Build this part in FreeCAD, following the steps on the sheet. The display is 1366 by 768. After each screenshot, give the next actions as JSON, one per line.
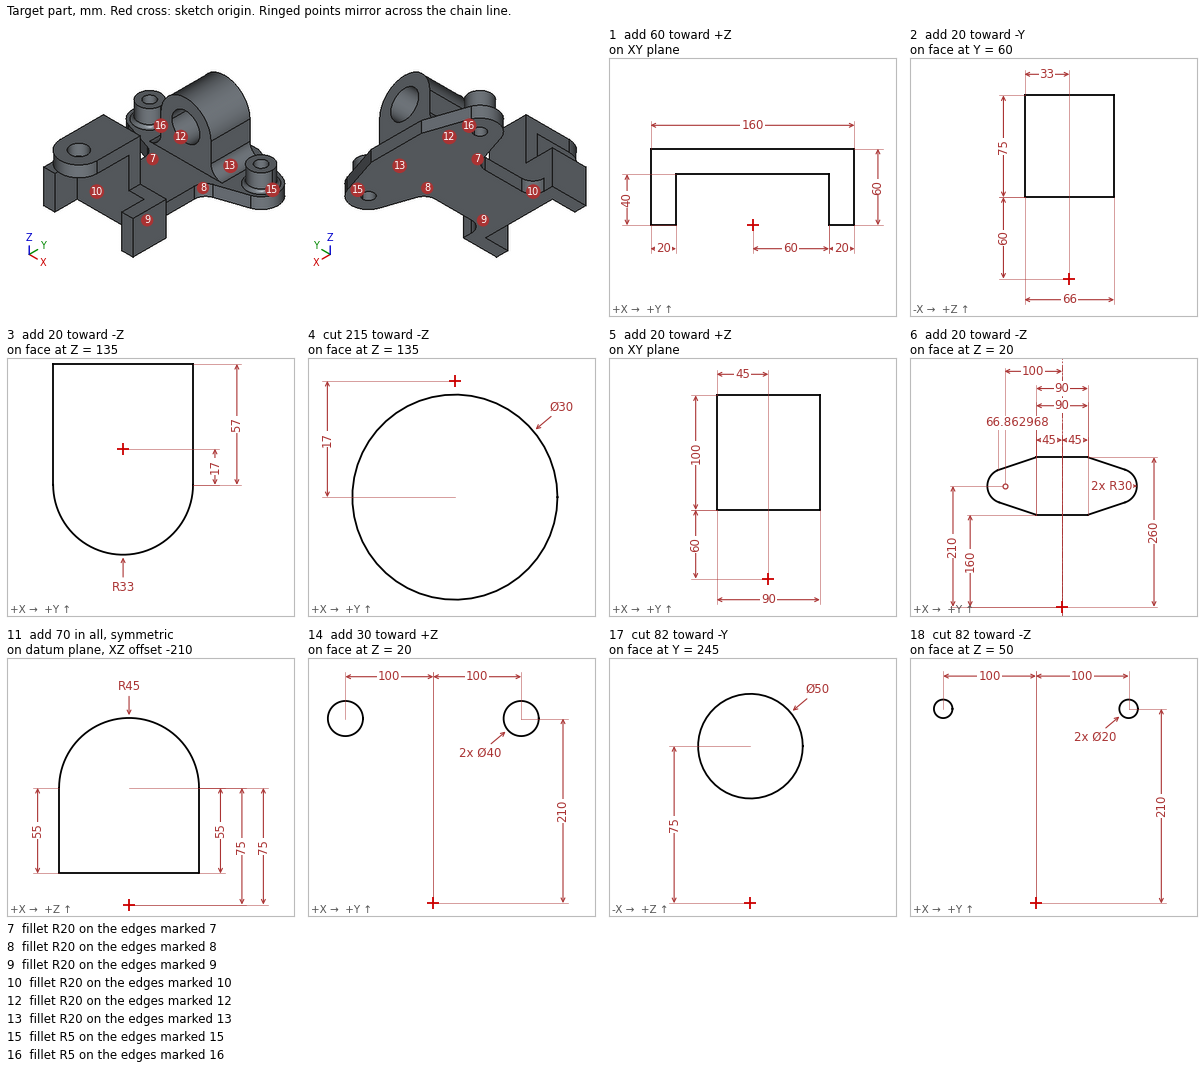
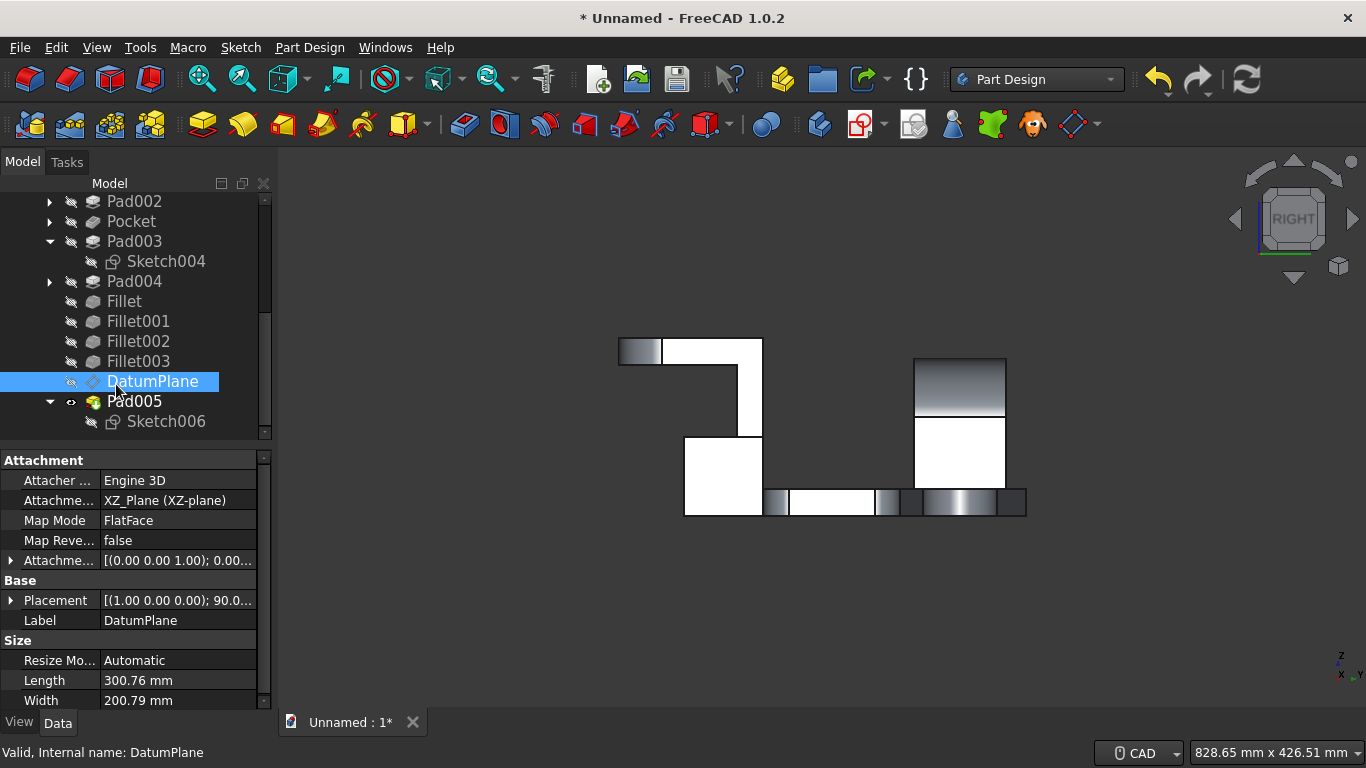
{"action": "key", "text": "v f"}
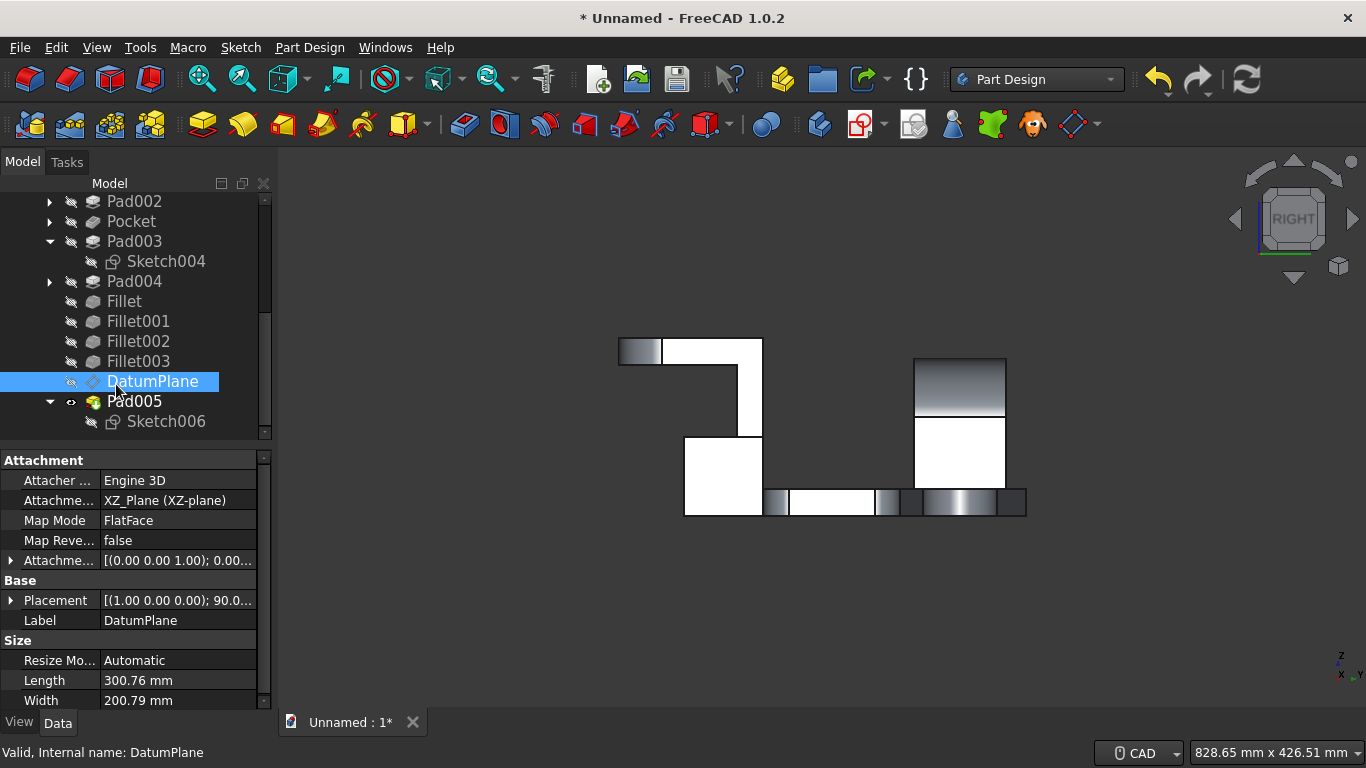
{"action": "key", "text": "5"}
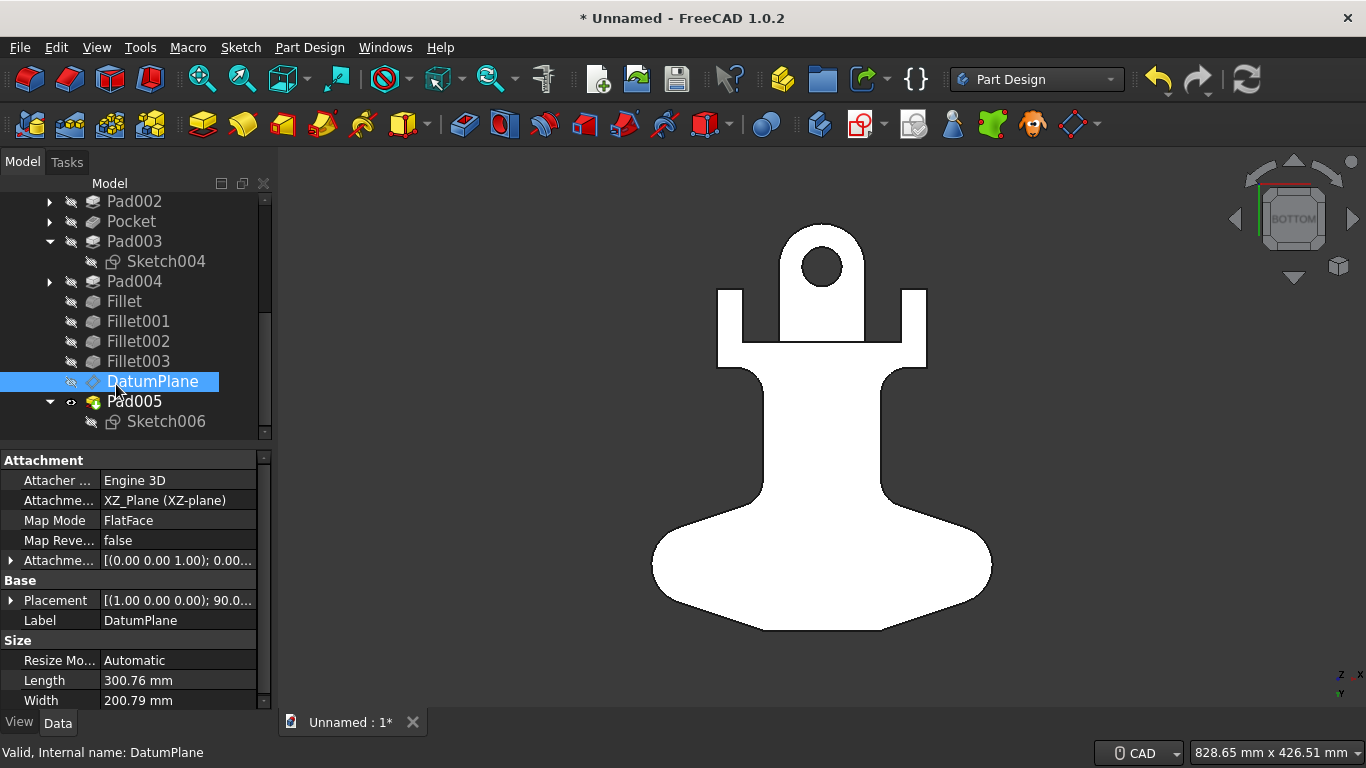
{"action": "key", "text": "4"}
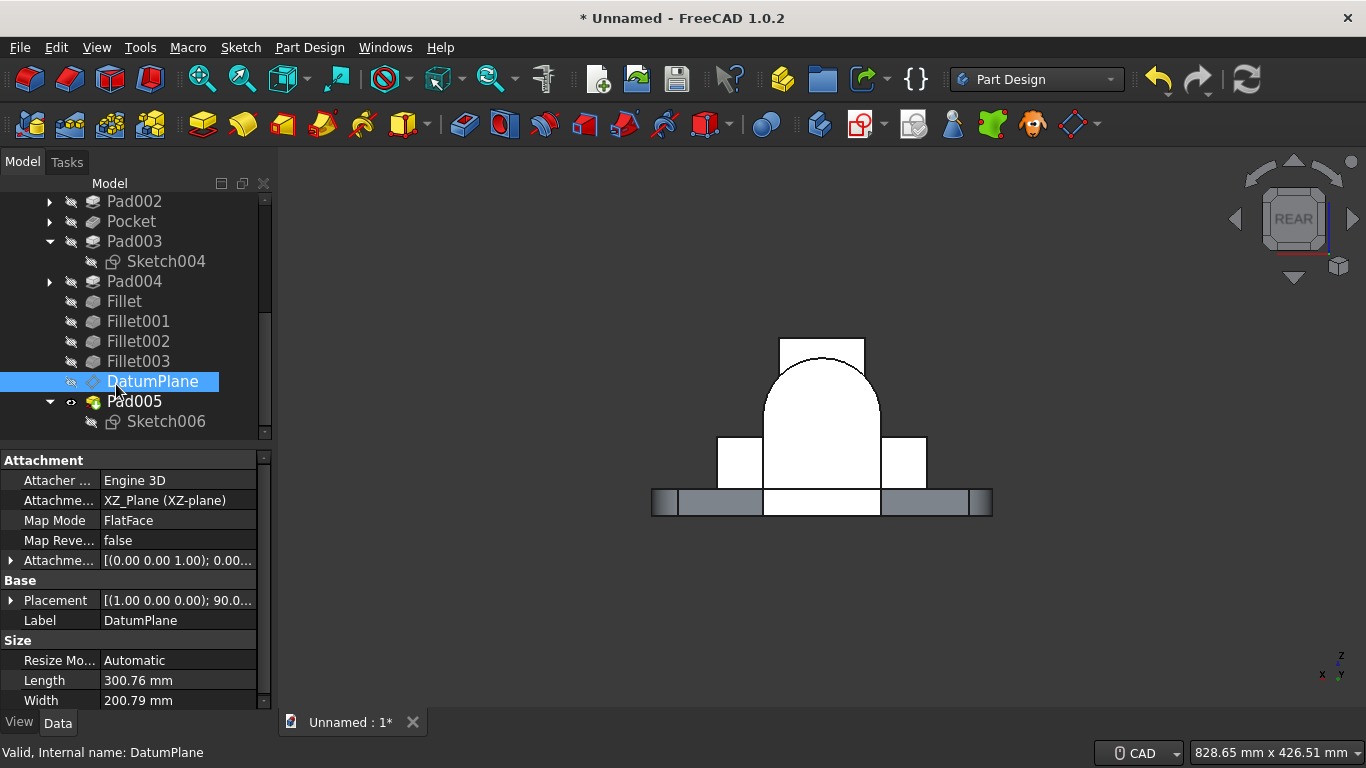
{"action": "left_click", "coordinate": [204, 80]}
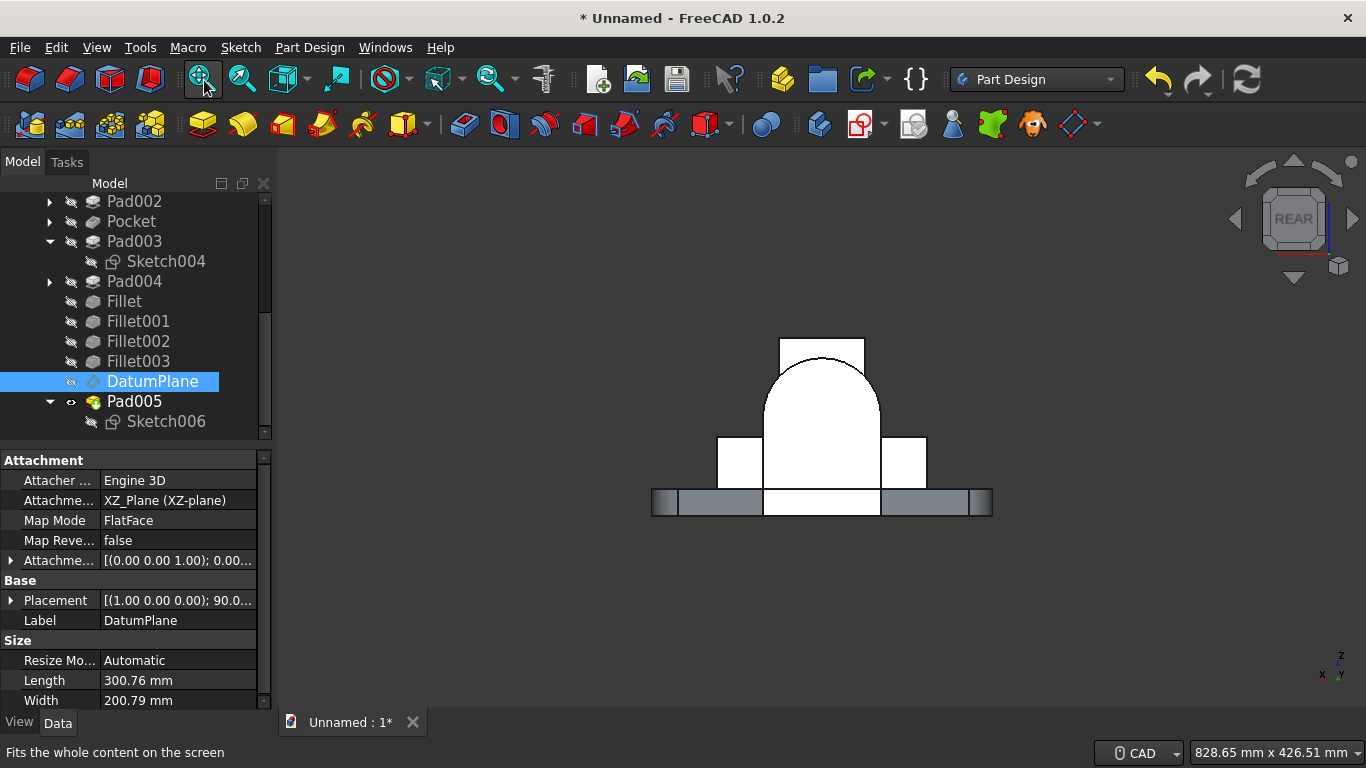
{"action": "key", "text": "6"}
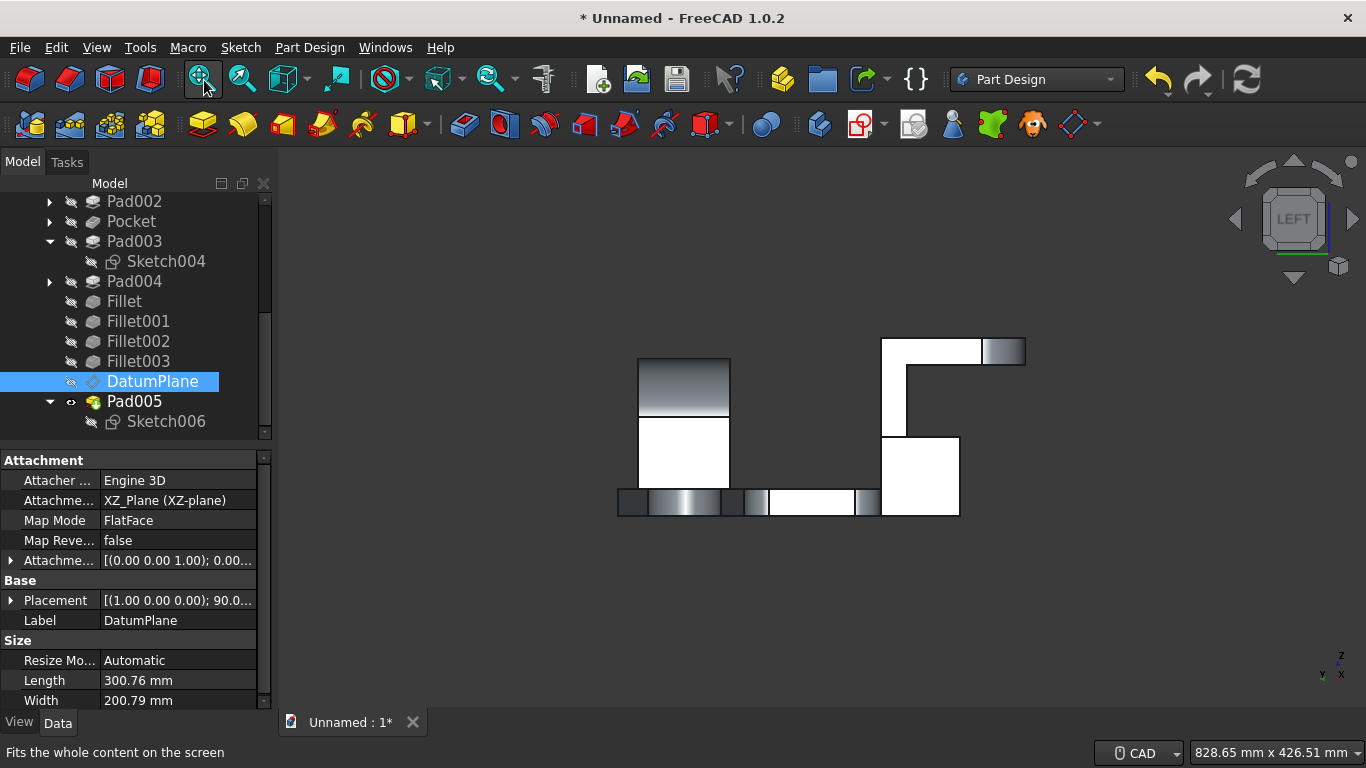
{"action": "key", "text": "v f"}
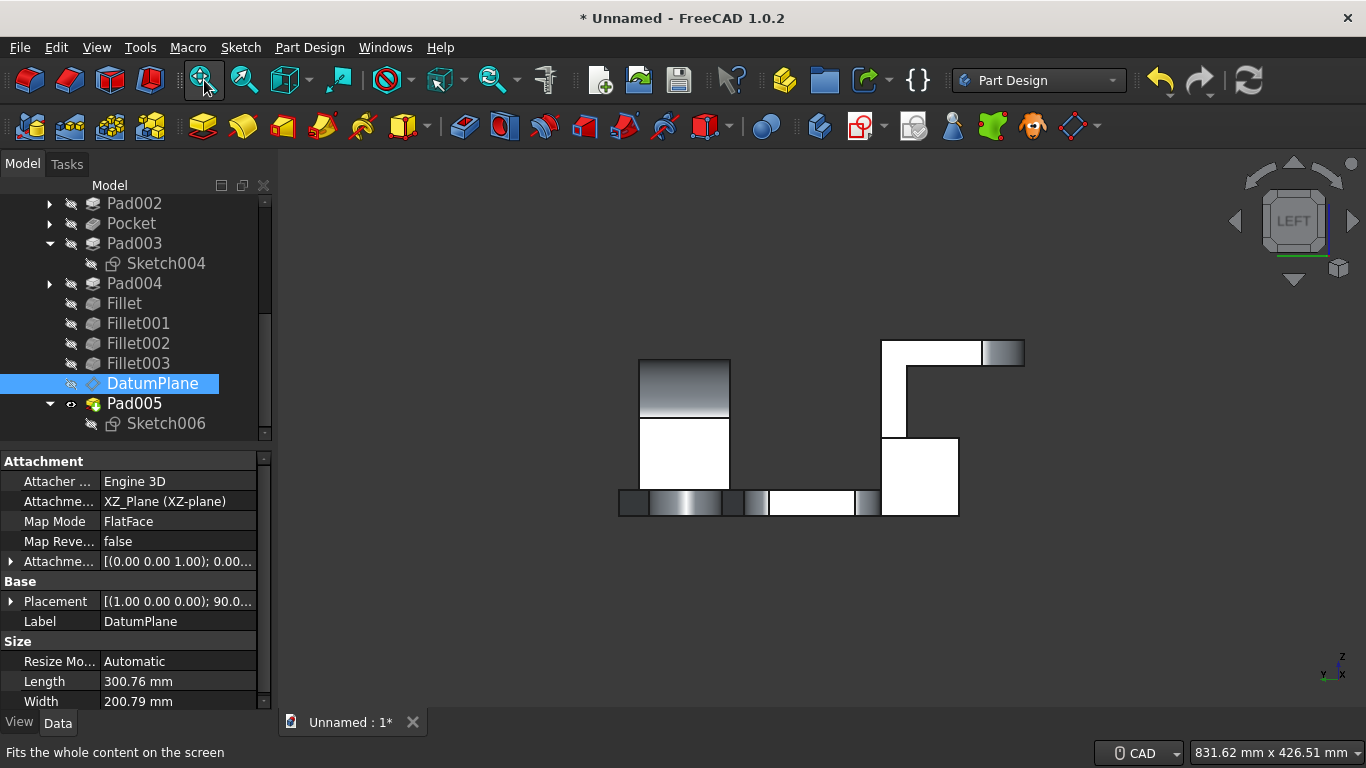
{"action": "key", "text": "v 3"}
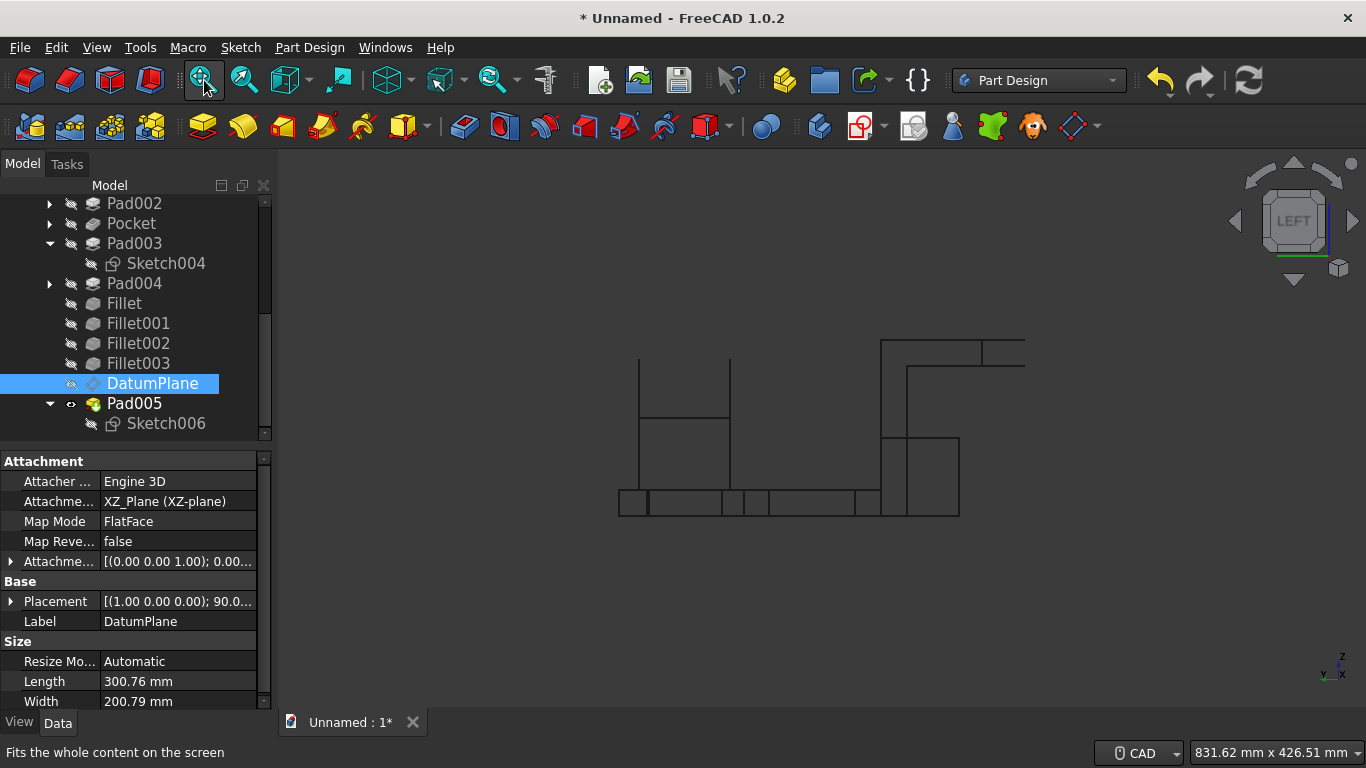
{"action": "key", "text": "0"}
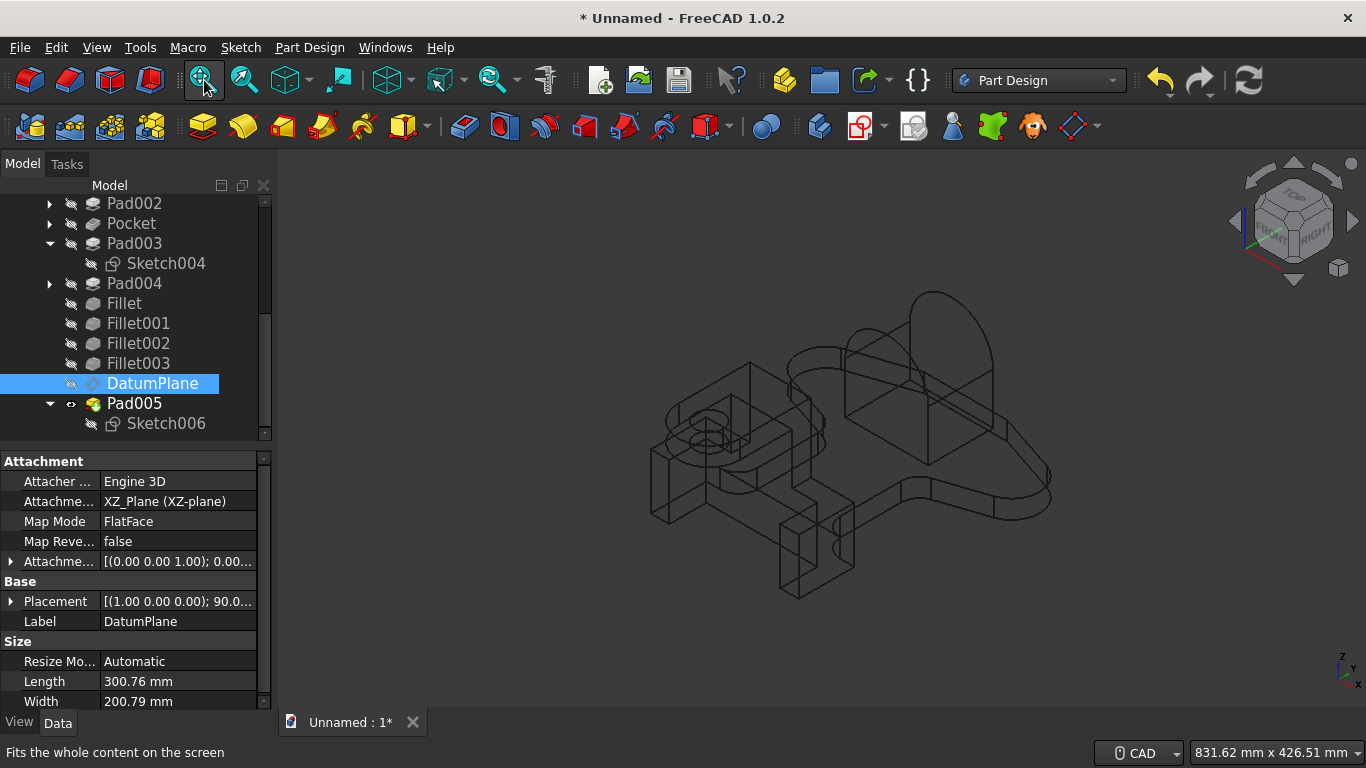
{"action": "left_click", "coordinate": [877, 398]}